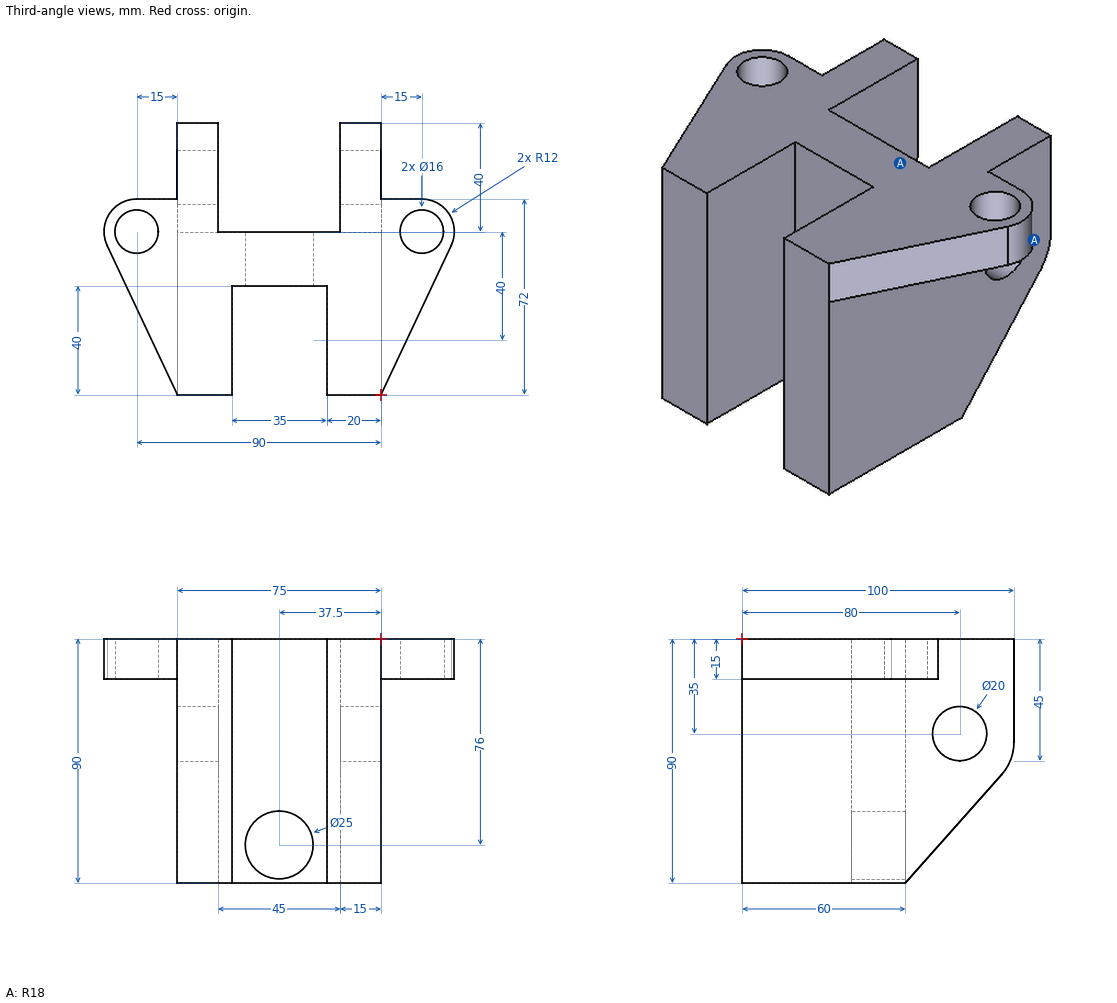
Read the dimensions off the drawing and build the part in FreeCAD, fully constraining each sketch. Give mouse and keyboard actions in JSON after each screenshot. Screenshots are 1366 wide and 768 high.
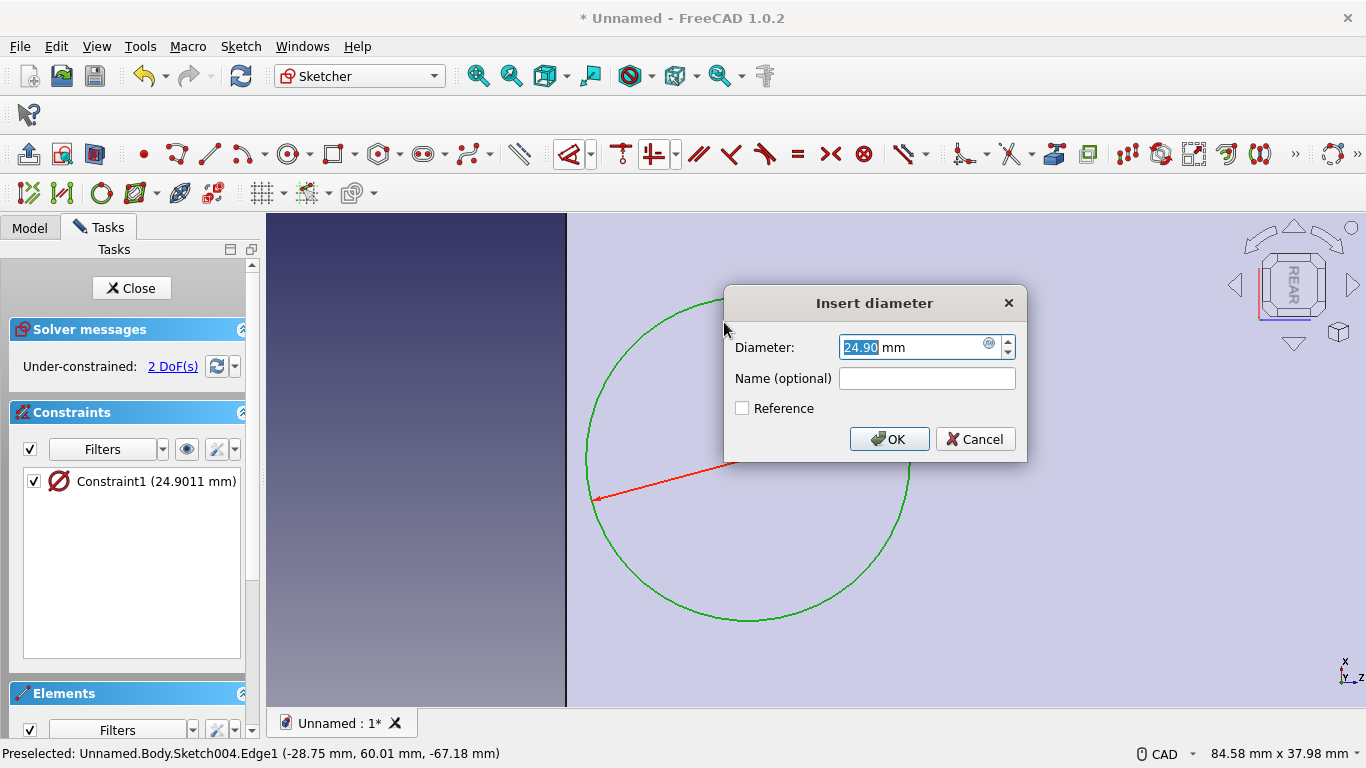
{"action": "type", "text": "25"}
{"action": "key", "text": "Return"}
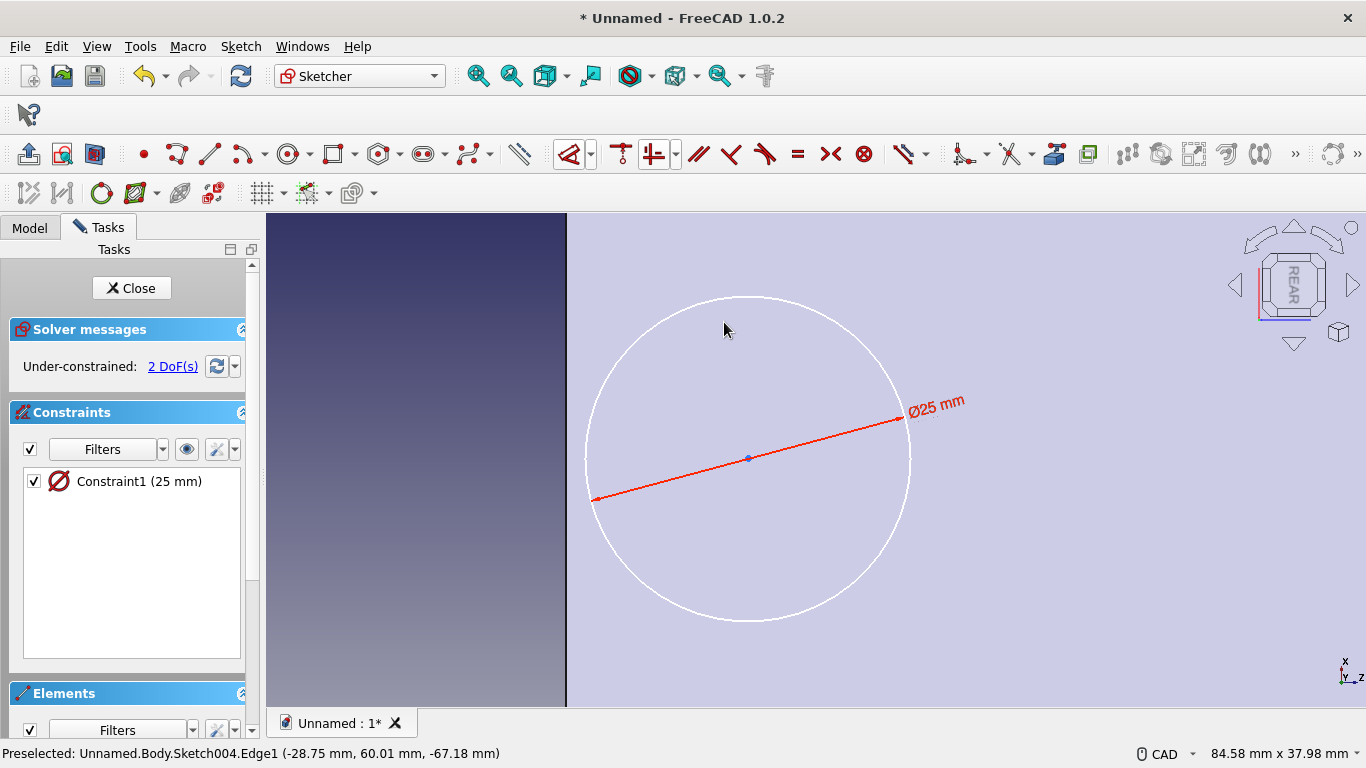
{"action": "left_click", "coordinate": [748, 459]}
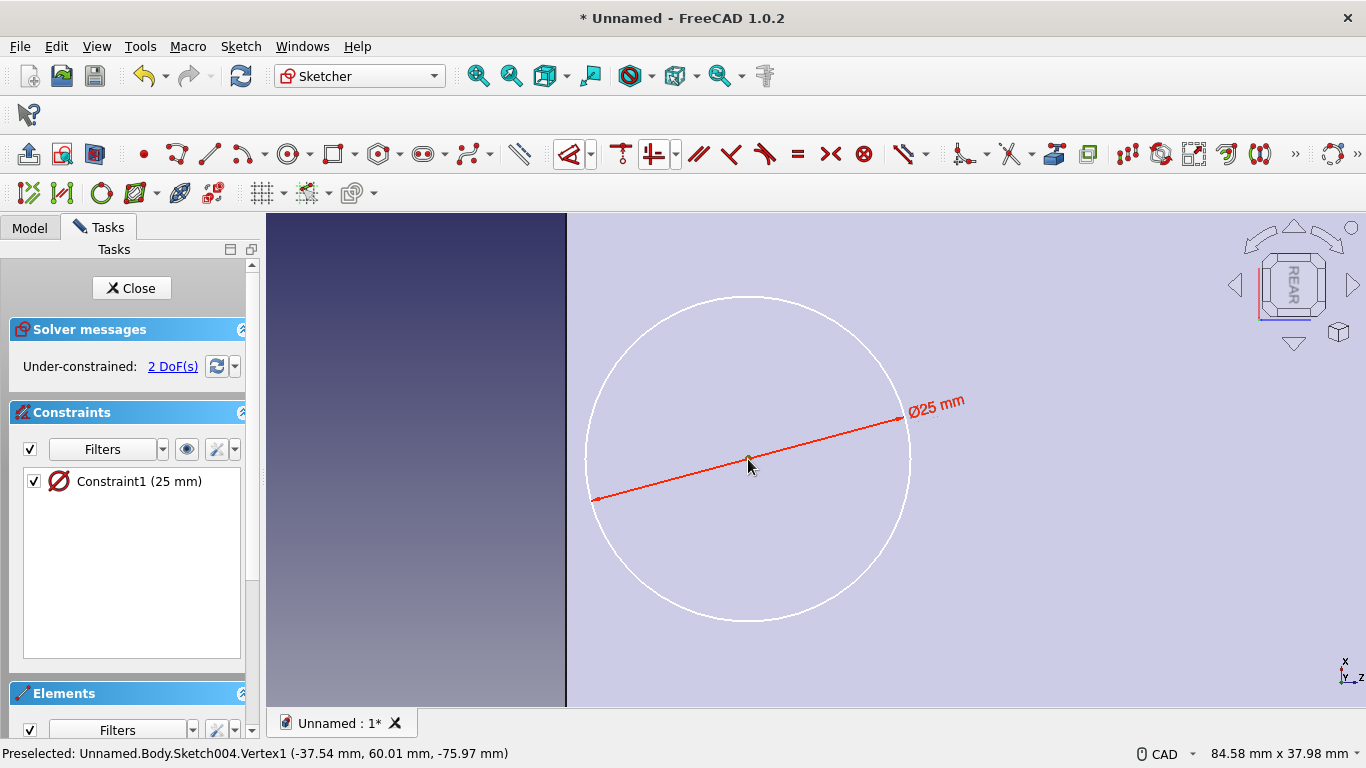
{"action": "left_click", "coordinate": [590, 154]}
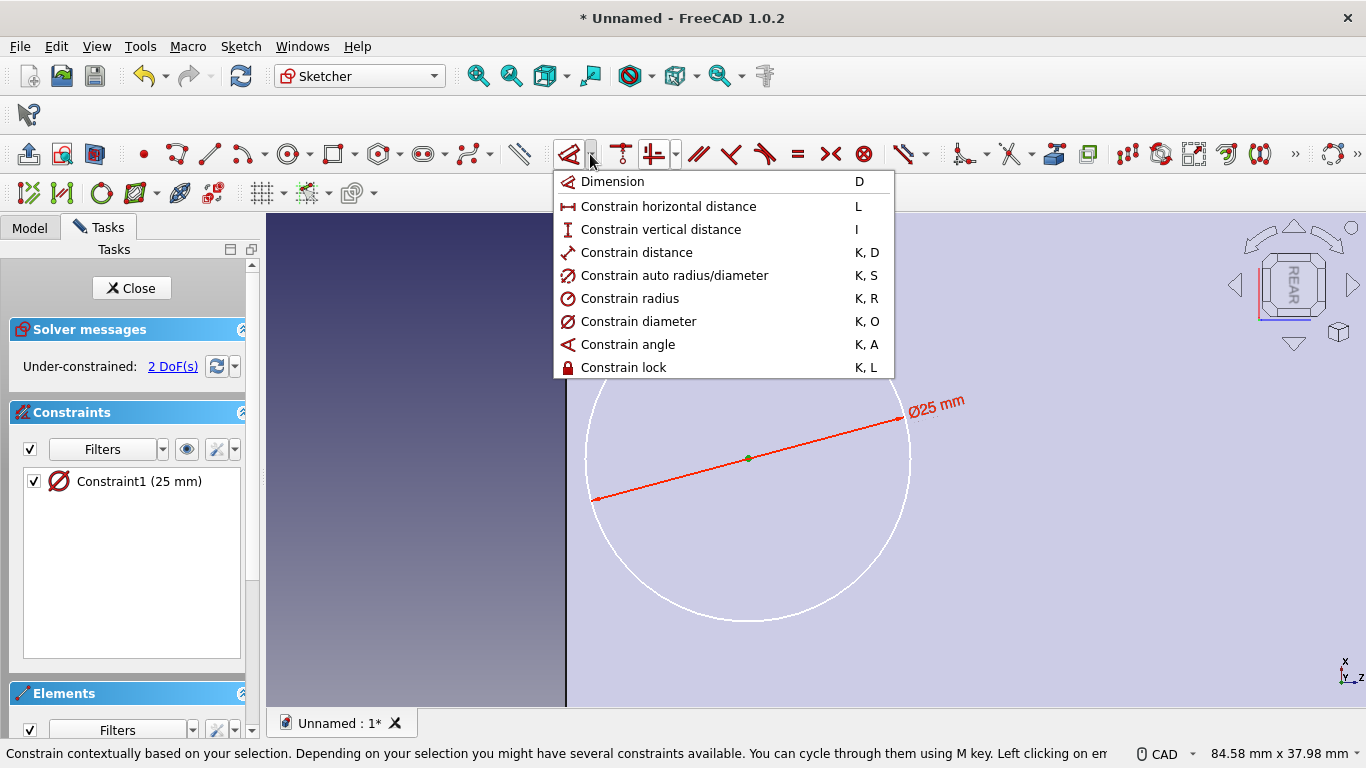
{"action": "left_click", "coordinate": [724, 206]}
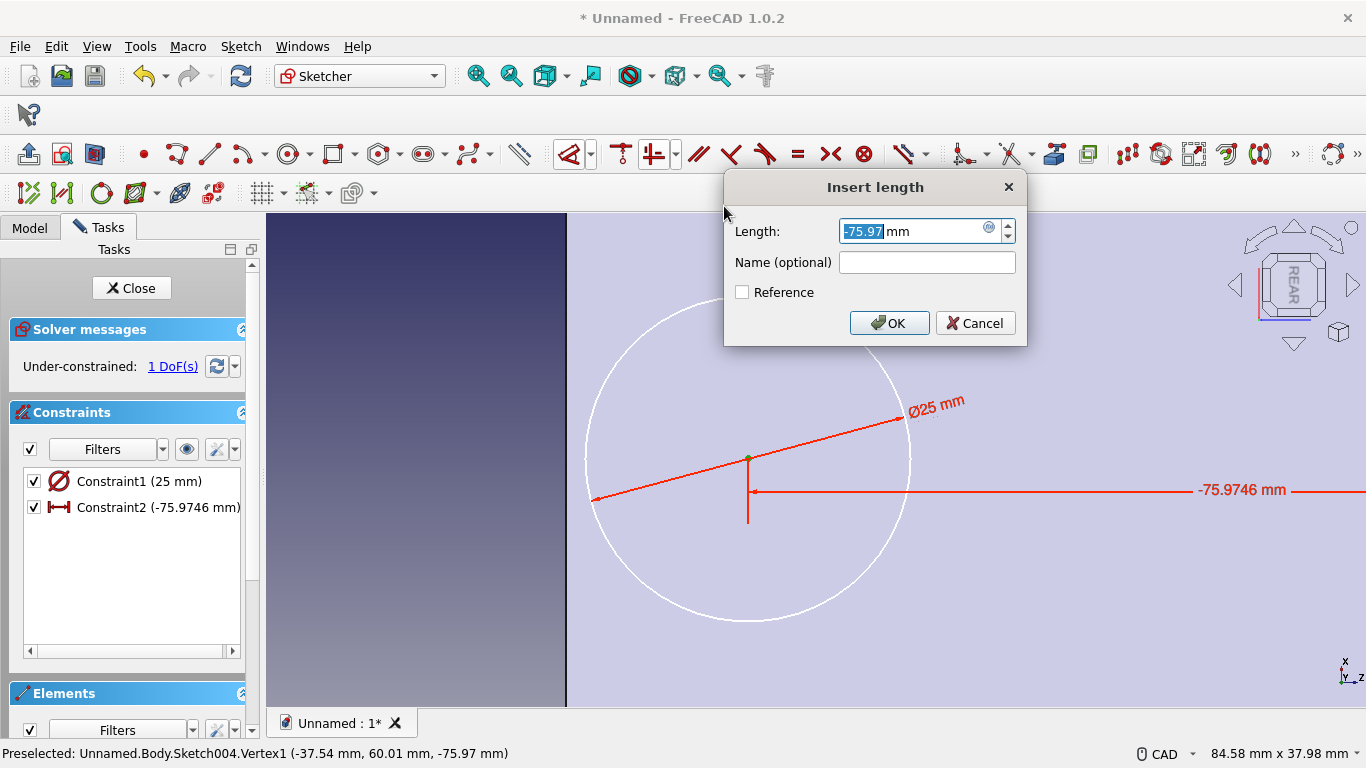
{"action": "type", "text": "-76"}
{"action": "key", "text": "Return"}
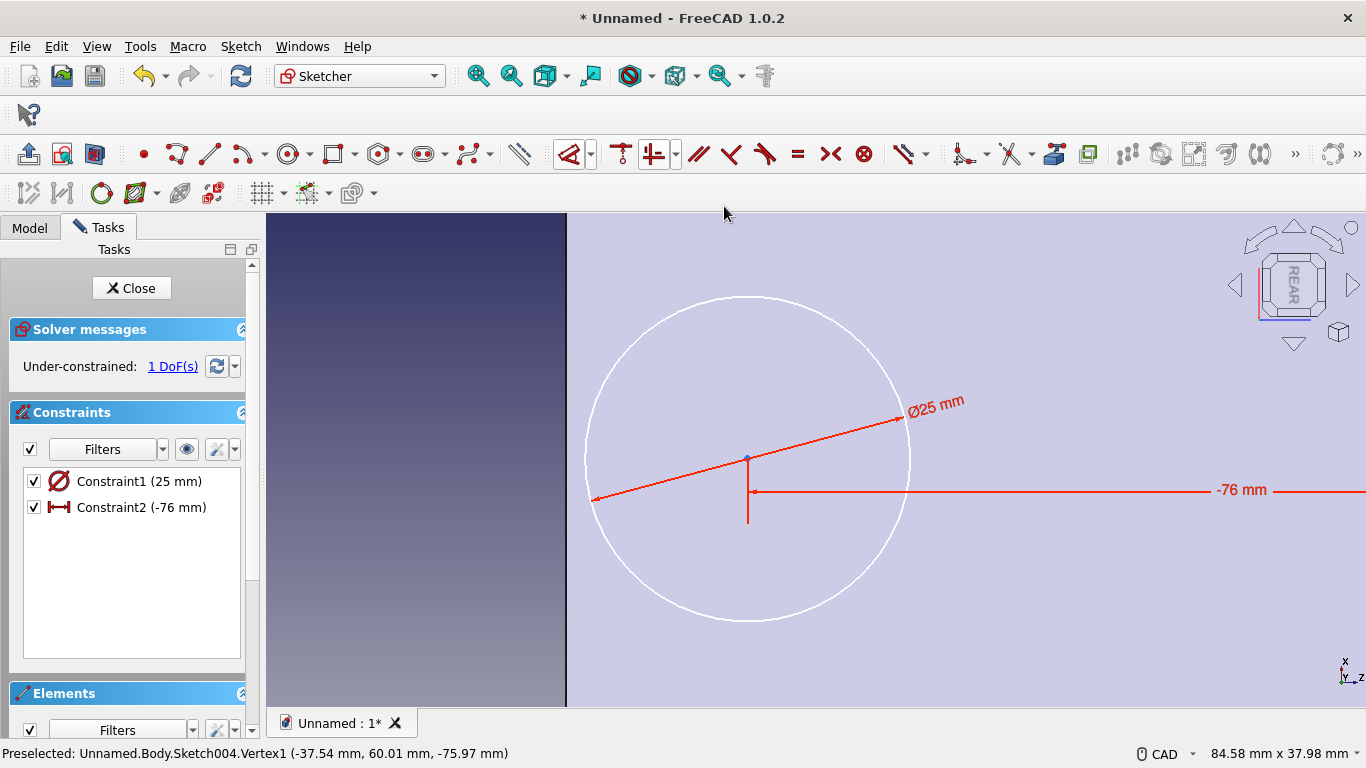
{"action": "left_click", "coordinate": [748, 459]}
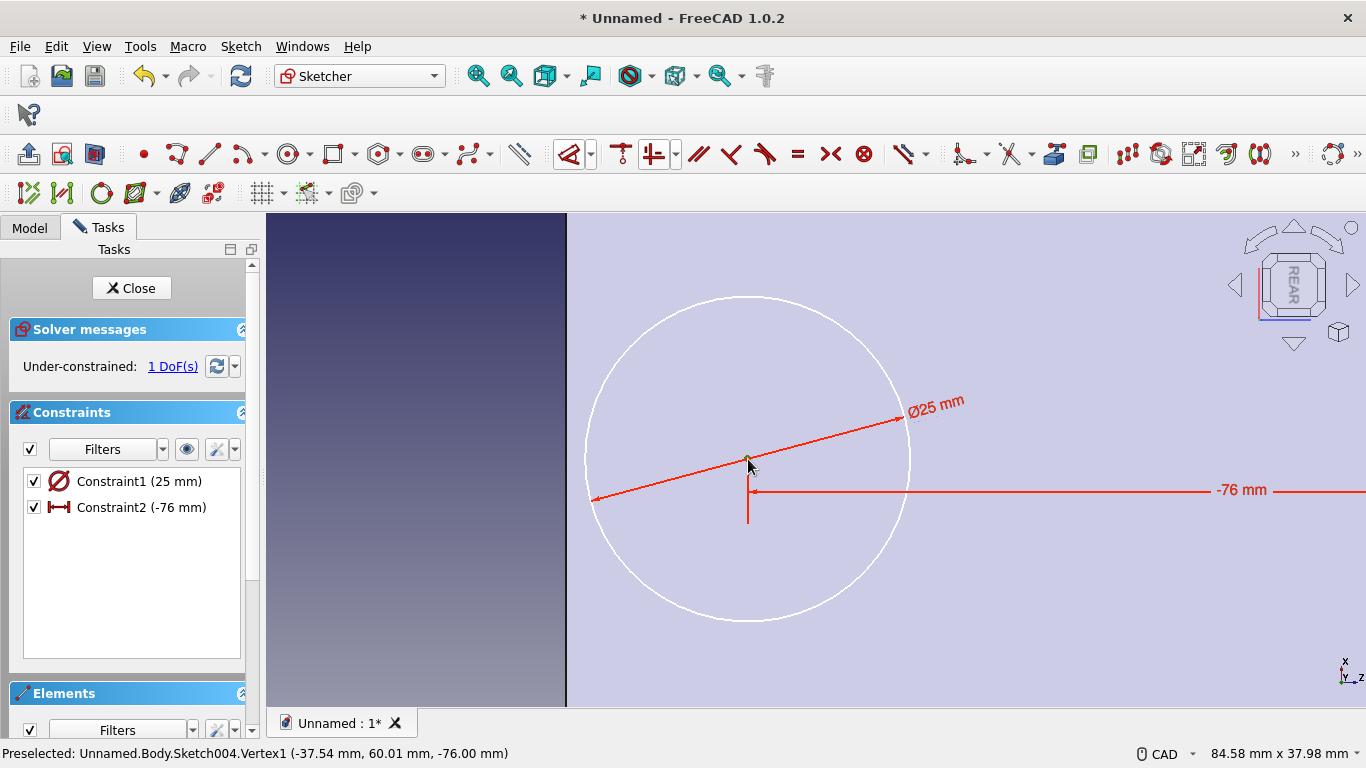
{"action": "left_click", "coordinate": [590, 154]}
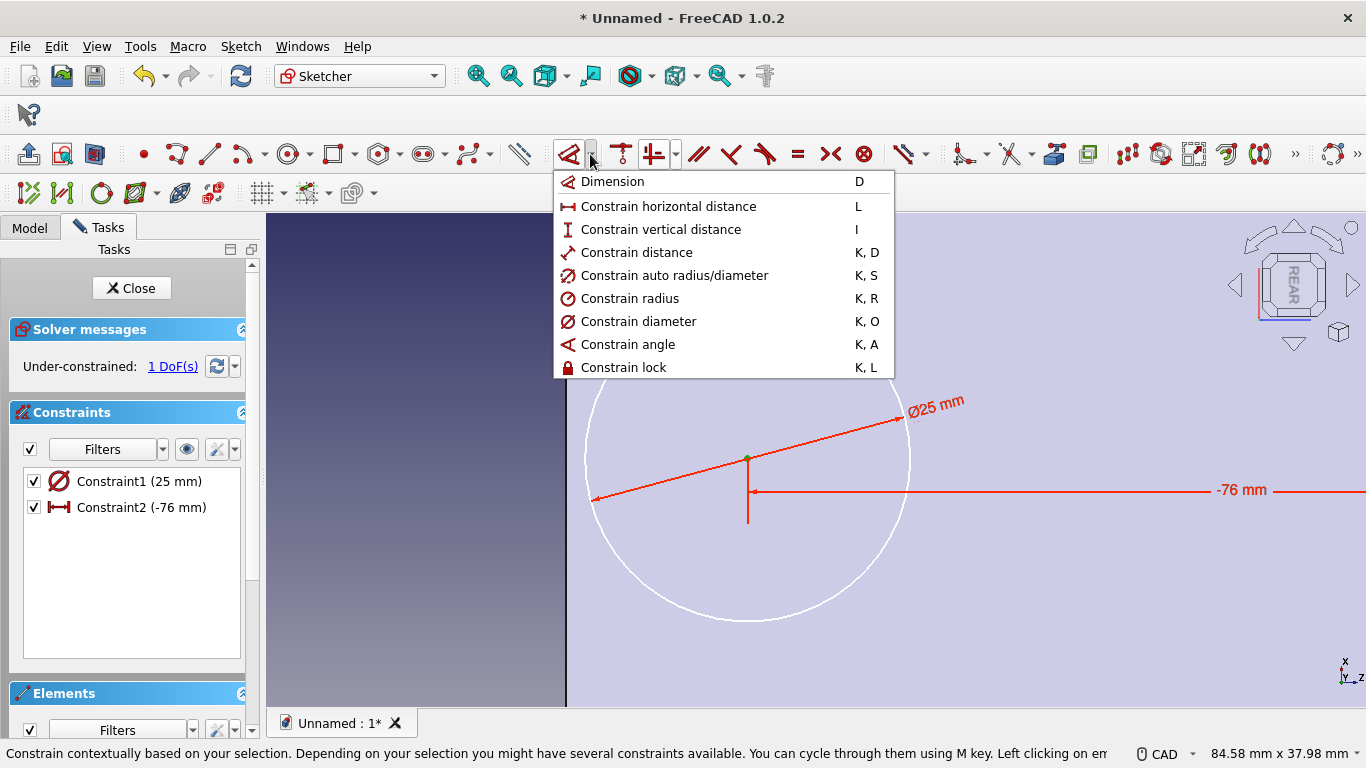
{"action": "left_click", "coordinate": [724, 230]}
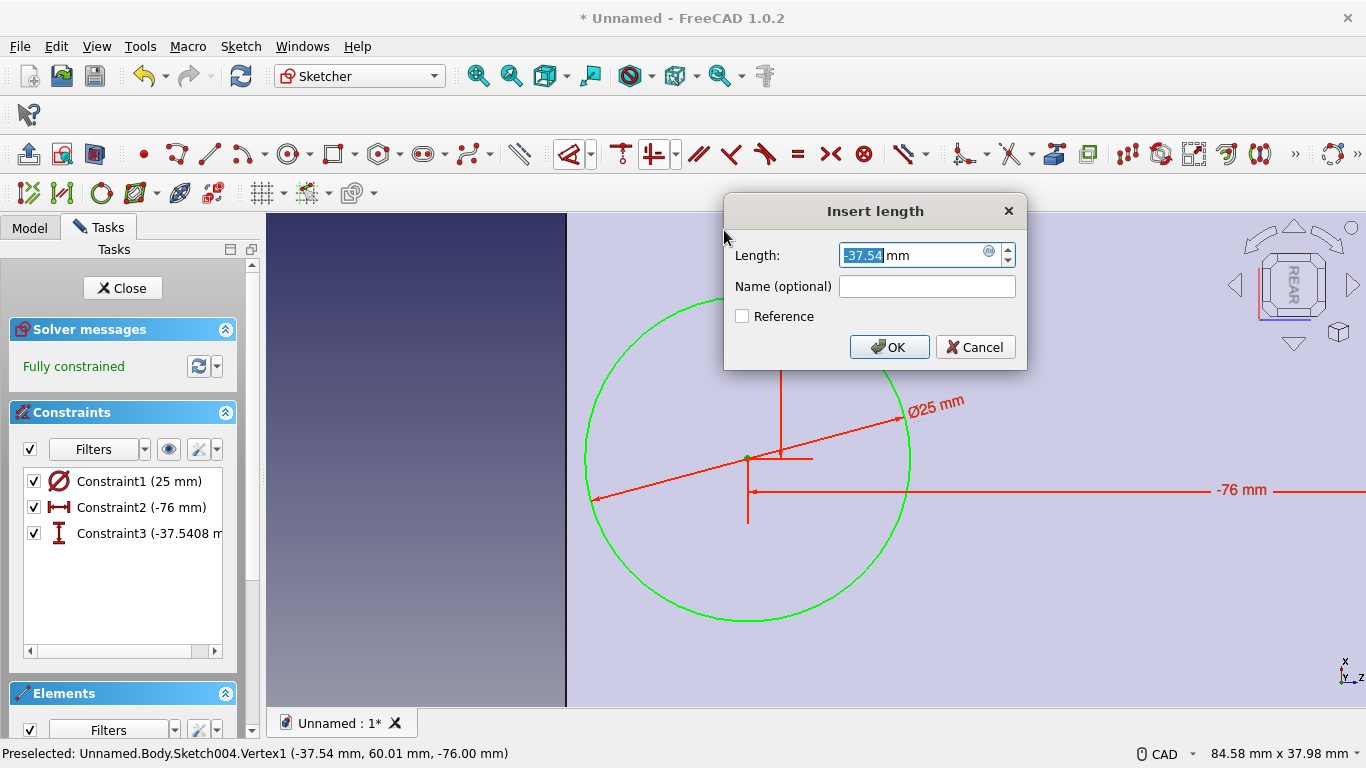
{"action": "type", "text": "-37.5"}
{"action": "key", "text": "Return"}